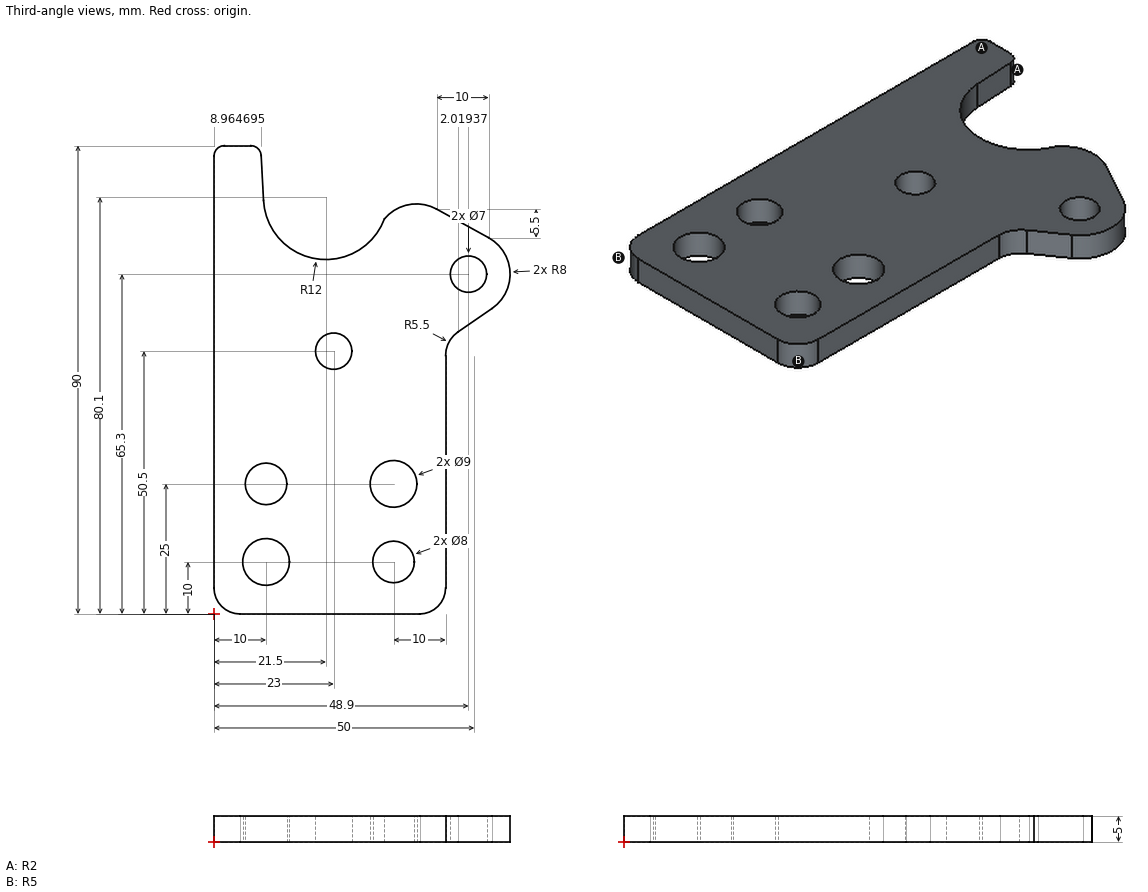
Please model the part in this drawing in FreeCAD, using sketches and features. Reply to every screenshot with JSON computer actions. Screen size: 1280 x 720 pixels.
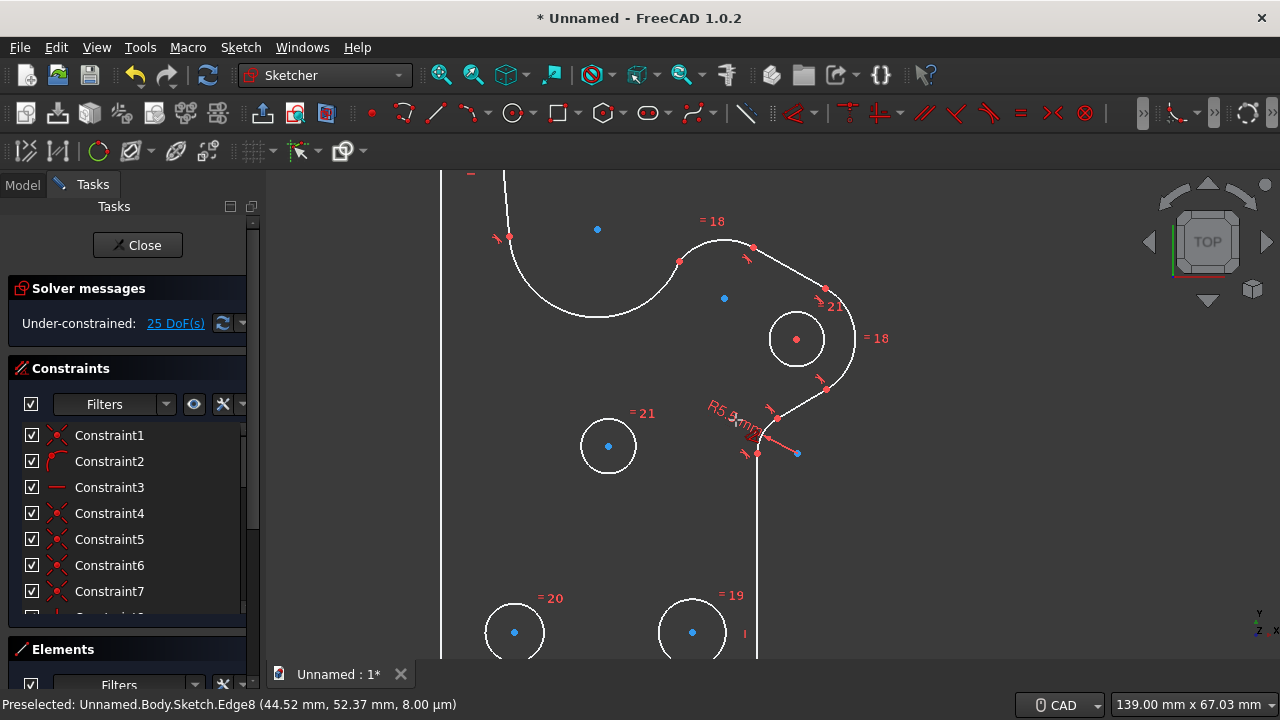
{"action": "left_click", "coordinate": [850, 362]}
{"action": "left_click", "coordinate": [879, 375]}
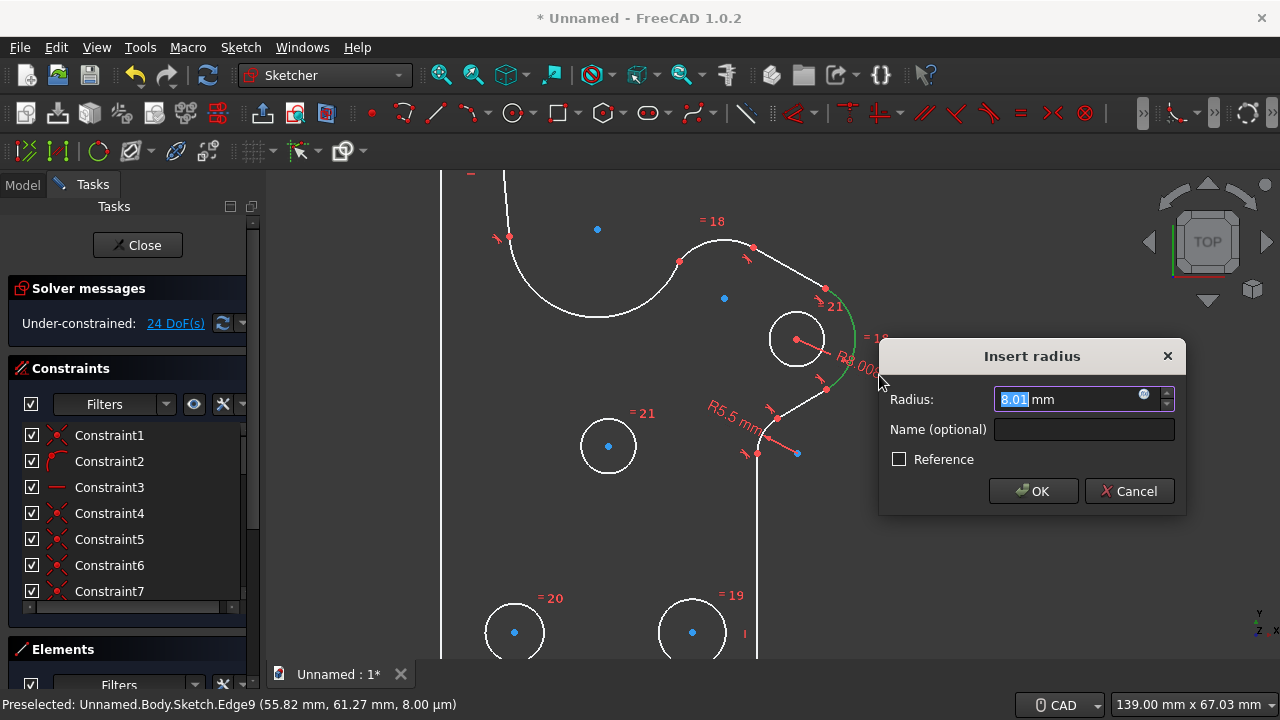
{"action": "type", "text": "8"}
{"action": "key", "text": "Return"}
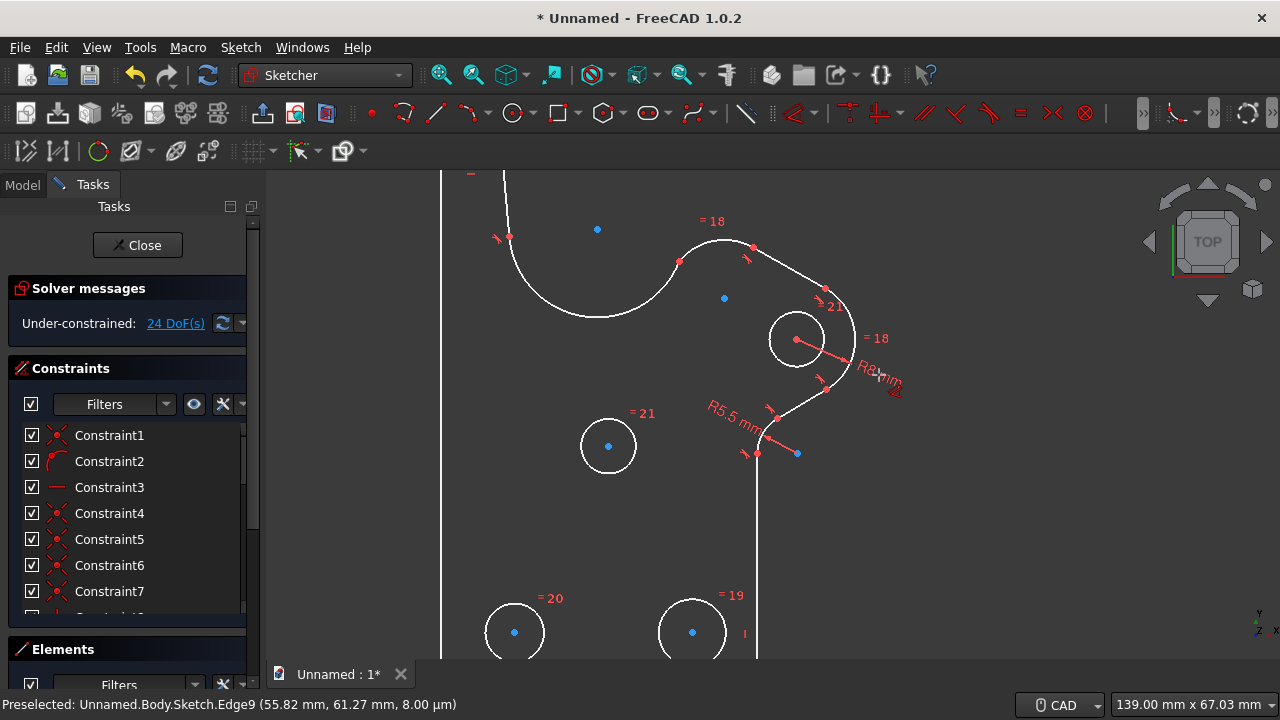
{"action": "left_click", "coordinate": [542, 298]}
{"action": "left_click", "coordinate": [522, 323]}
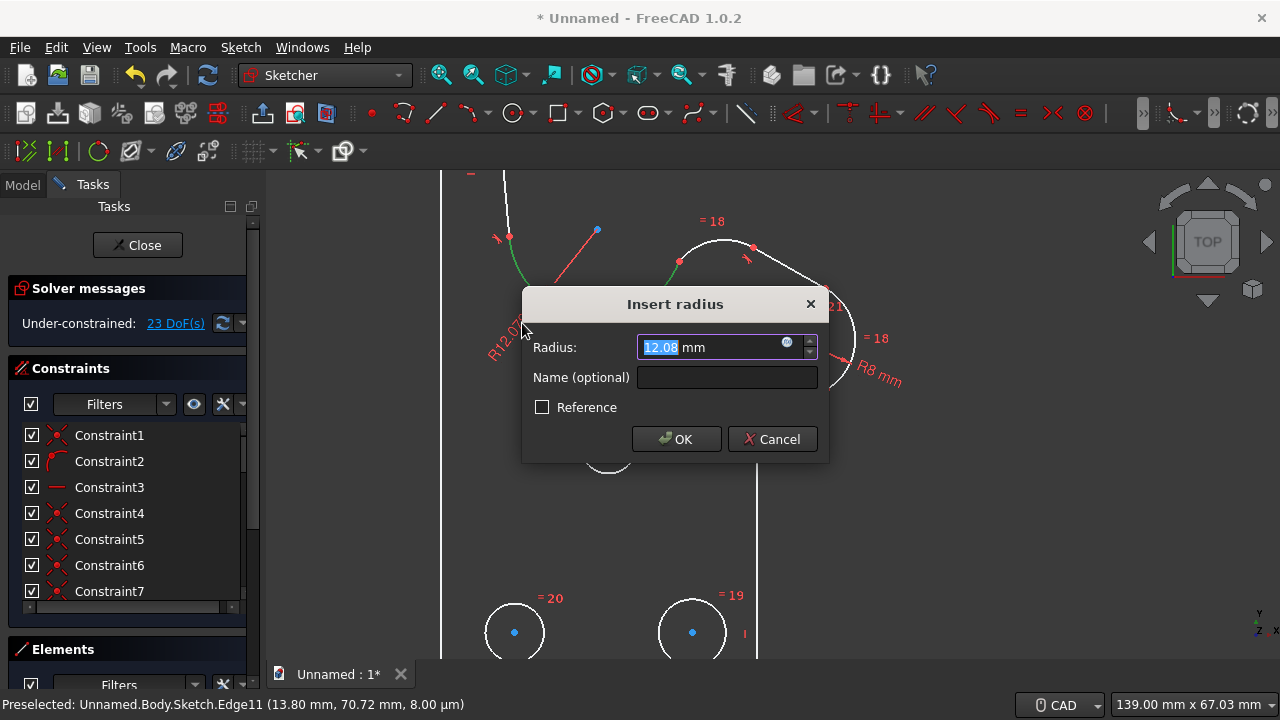
{"action": "type", "text": "12"}
{"action": "key", "text": "Return"}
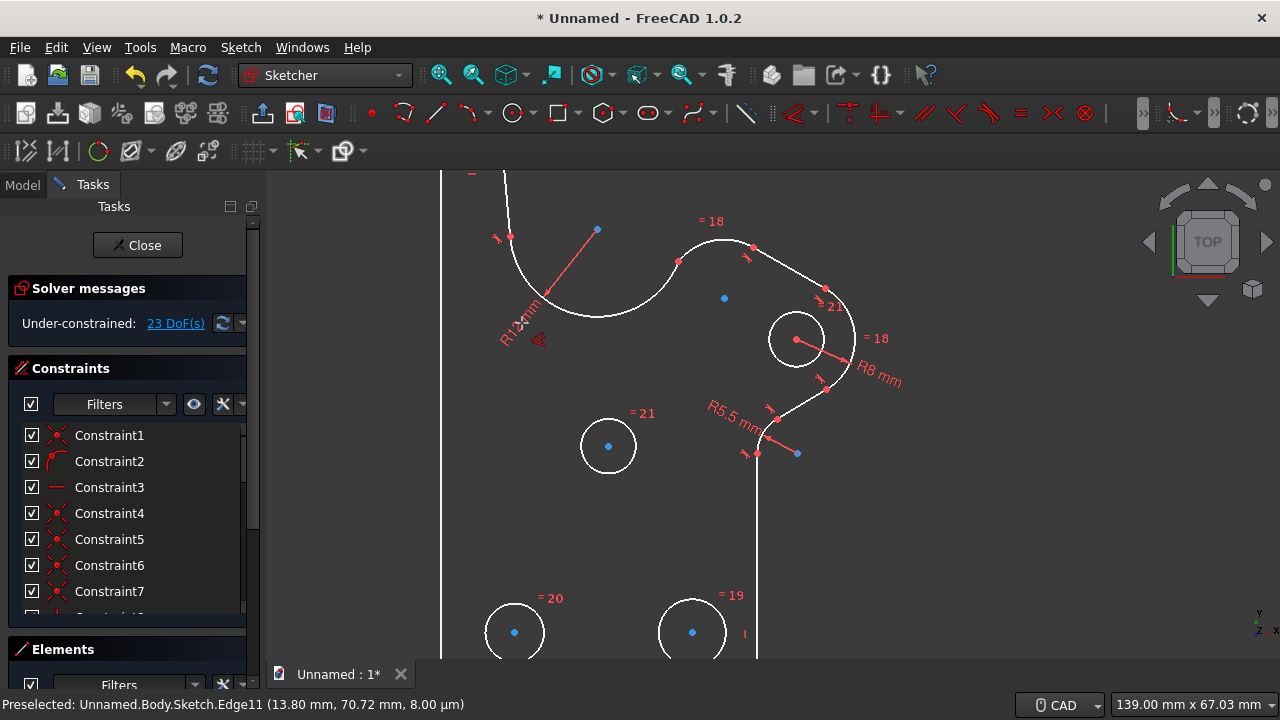
{"action": "scroll", "coordinate": [750, 357], "scroll_direction": "down", "scroll_amount": 4}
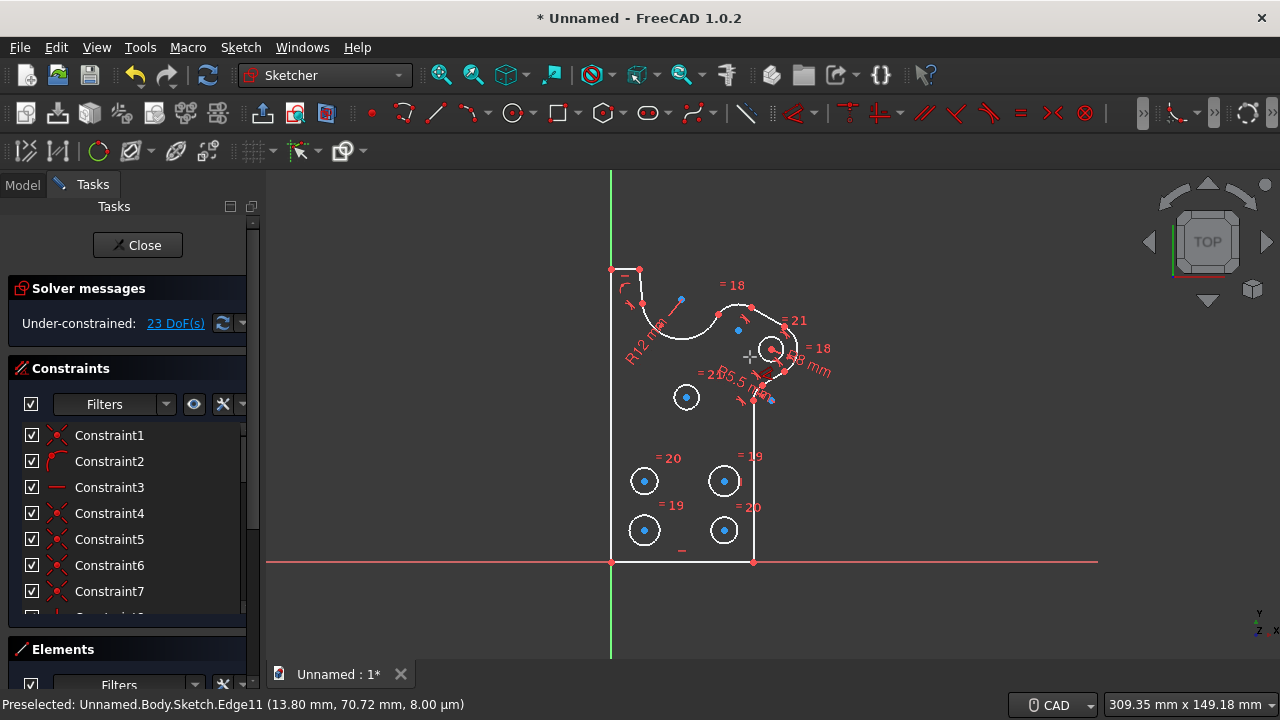
{"action": "scroll", "coordinate": [734, 521], "scroll_direction": "up", "scroll_amount": 3}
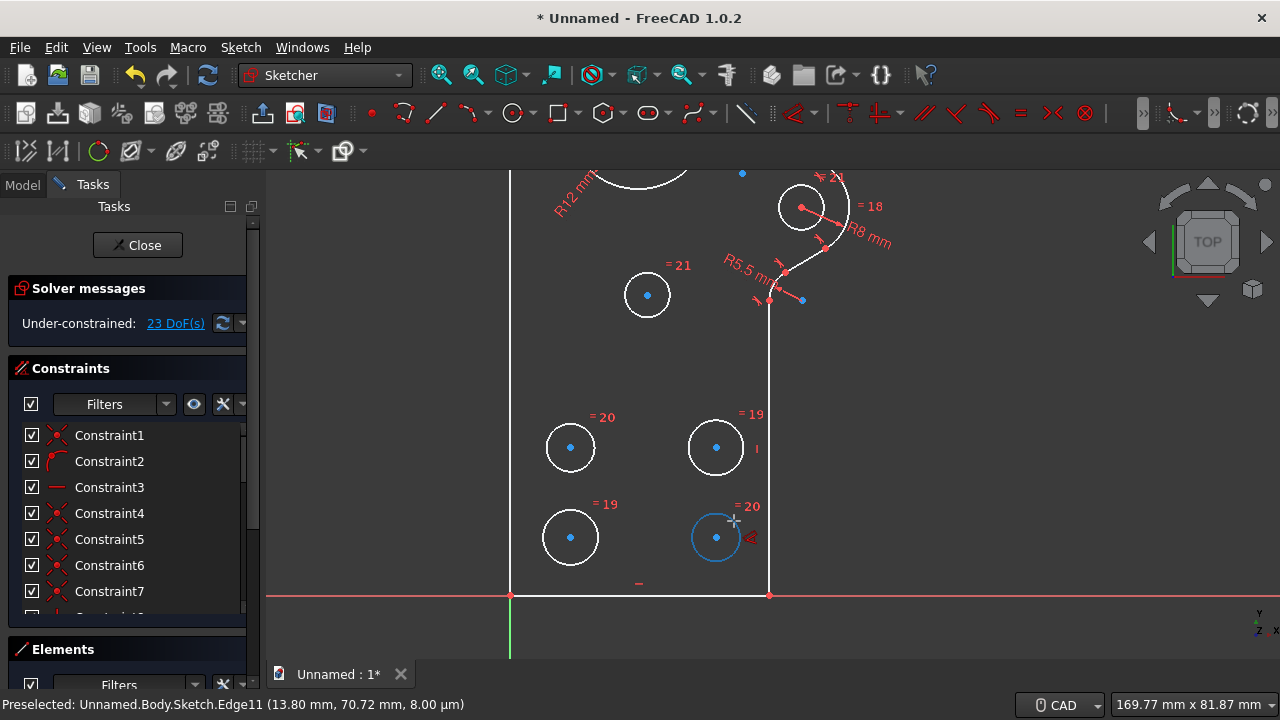
{"action": "left_click", "coordinate": [733, 520]}
{"action": "left_click", "coordinate": [755, 497]}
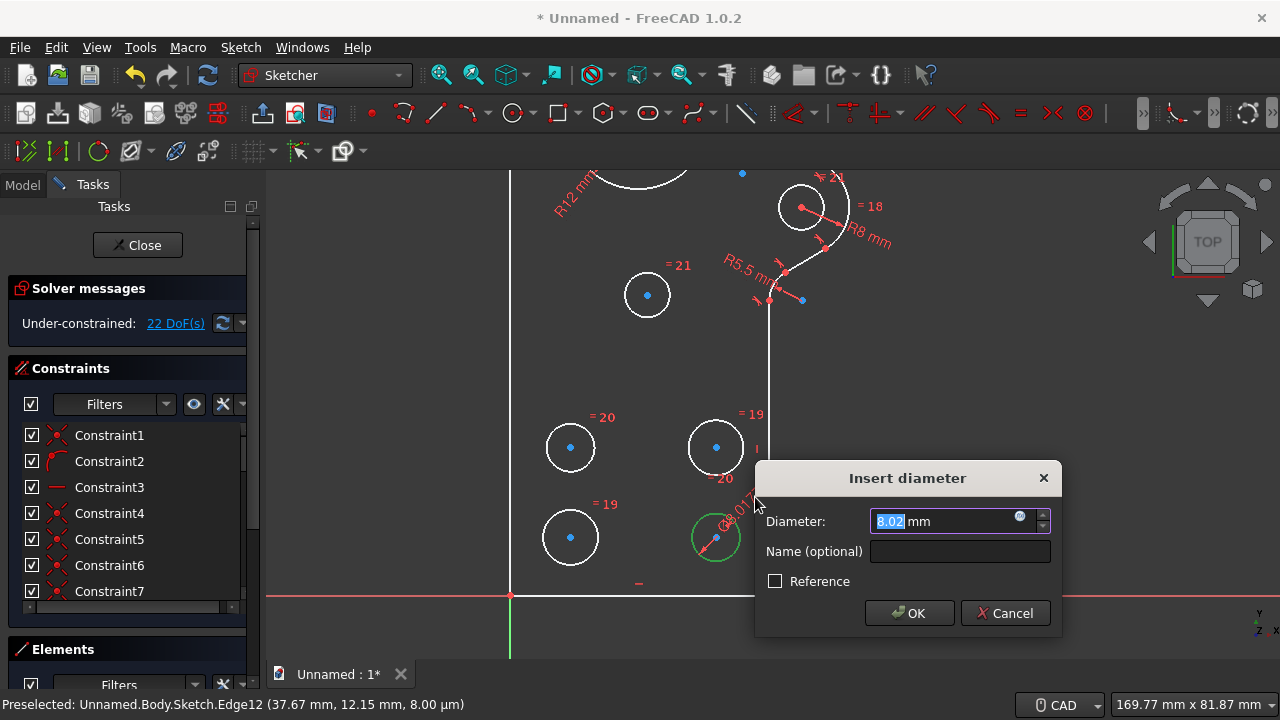
{"action": "type", "text": "8"}
{"action": "key", "text": "Return"}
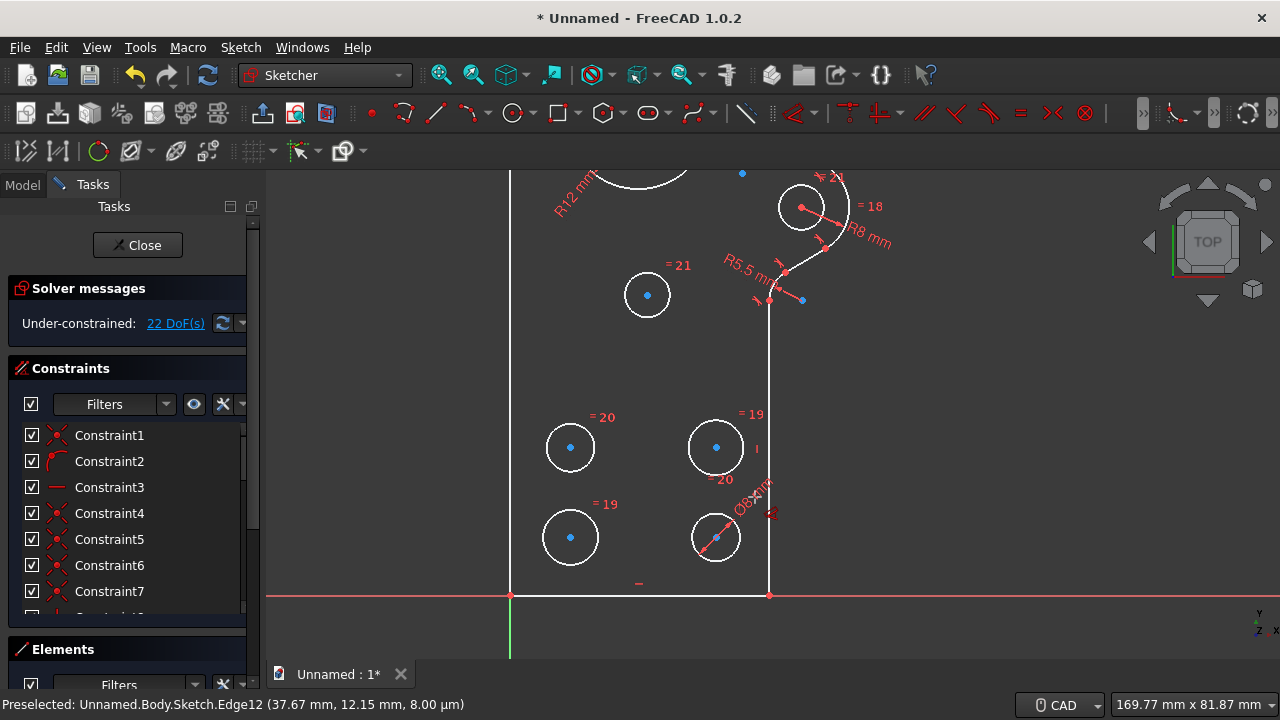
{"action": "left_click", "coordinate": [735, 428]}
{"action": "left_click", "coordinate": [732, 390]}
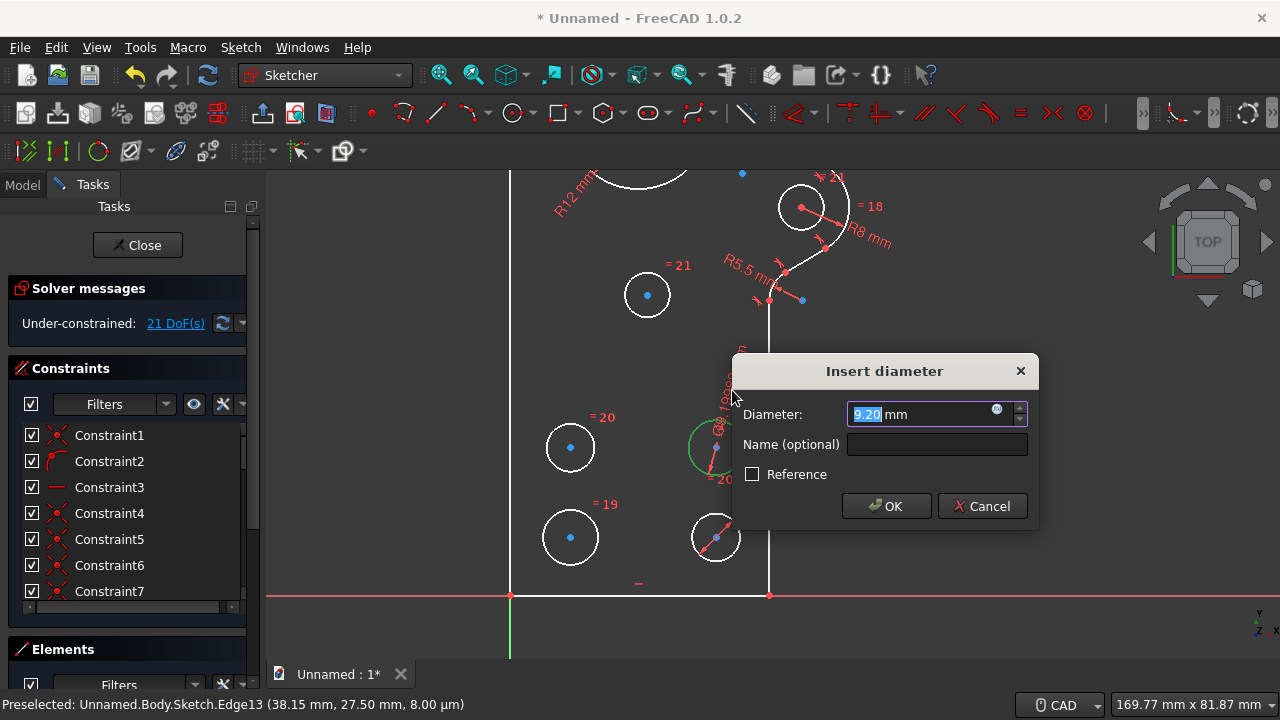
{"action": "type", "text": "9"}
{"action": "key", "text": "Return"}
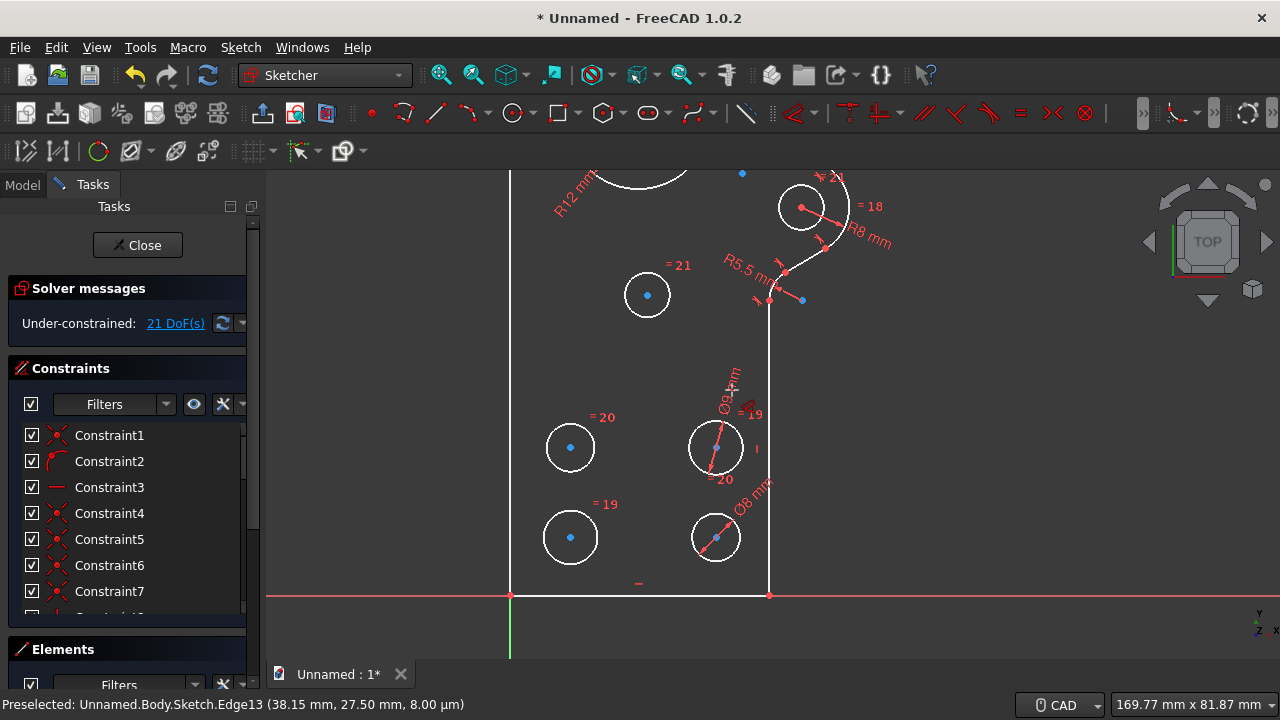
{"action": "left_click", "coordinate": [786, 223]}
{"action": "left_click", "coordinate": [763, 246]}